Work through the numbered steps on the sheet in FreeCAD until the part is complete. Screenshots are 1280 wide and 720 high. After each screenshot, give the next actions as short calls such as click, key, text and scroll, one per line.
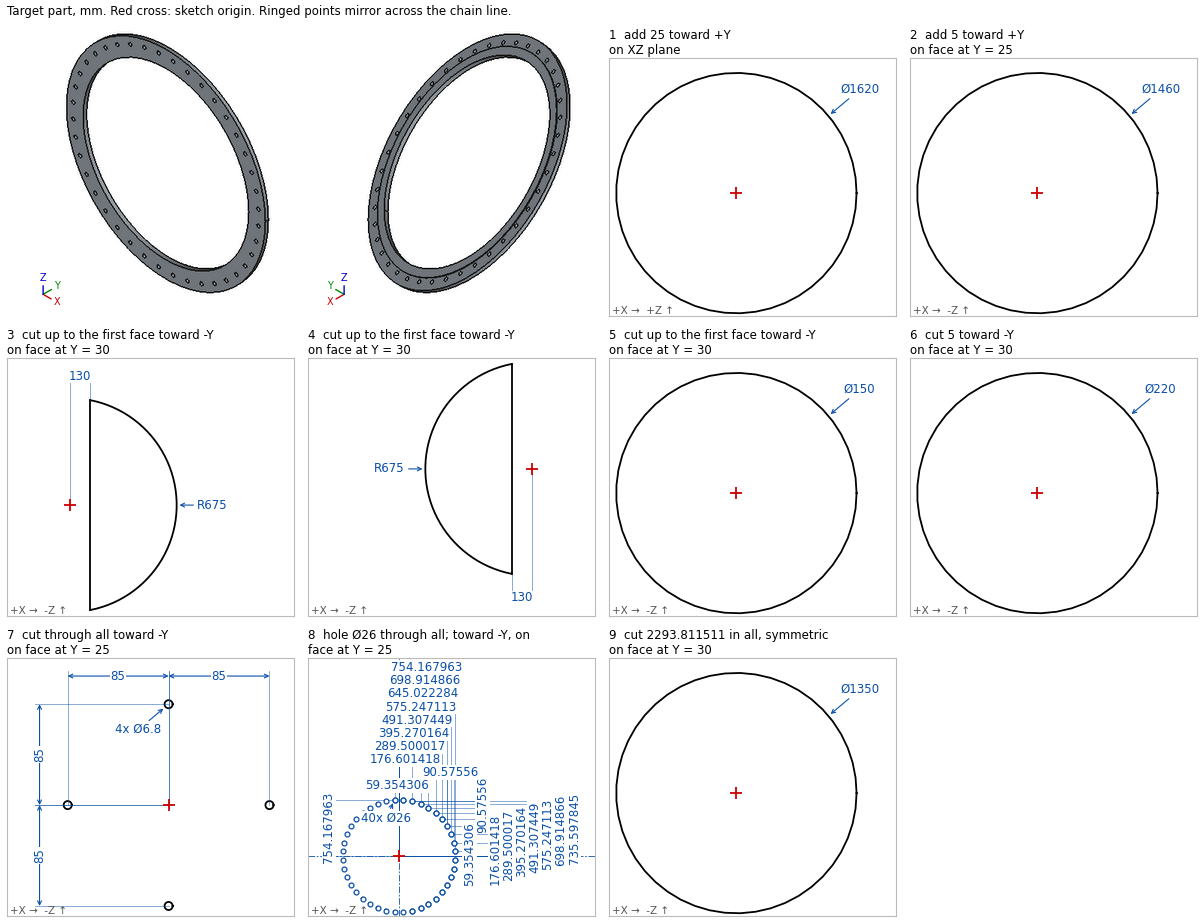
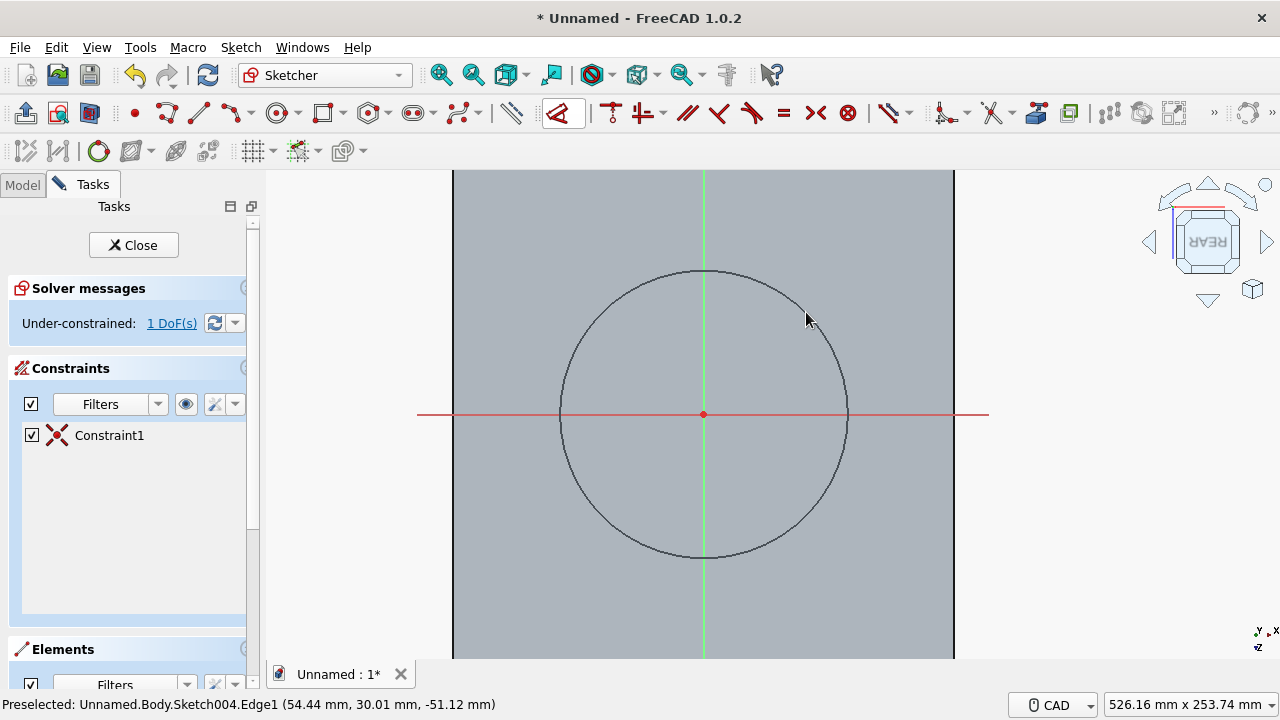
click(805, 312)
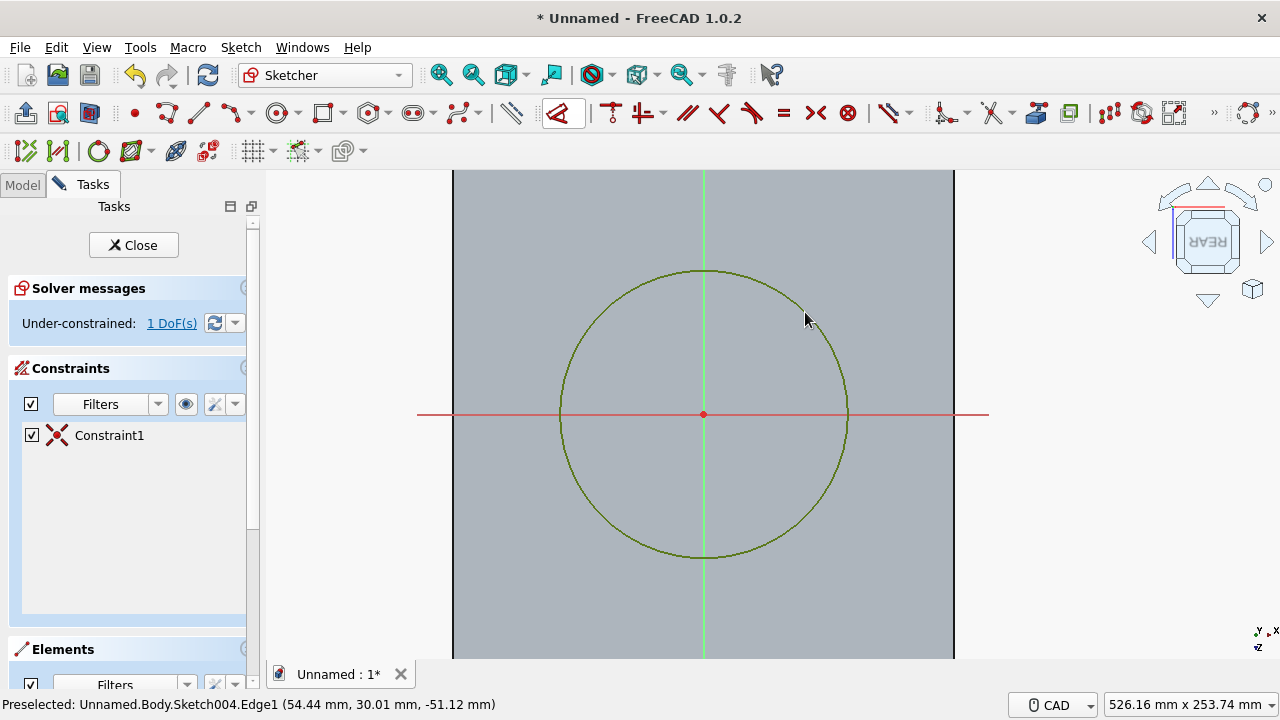
key(k)
key(o)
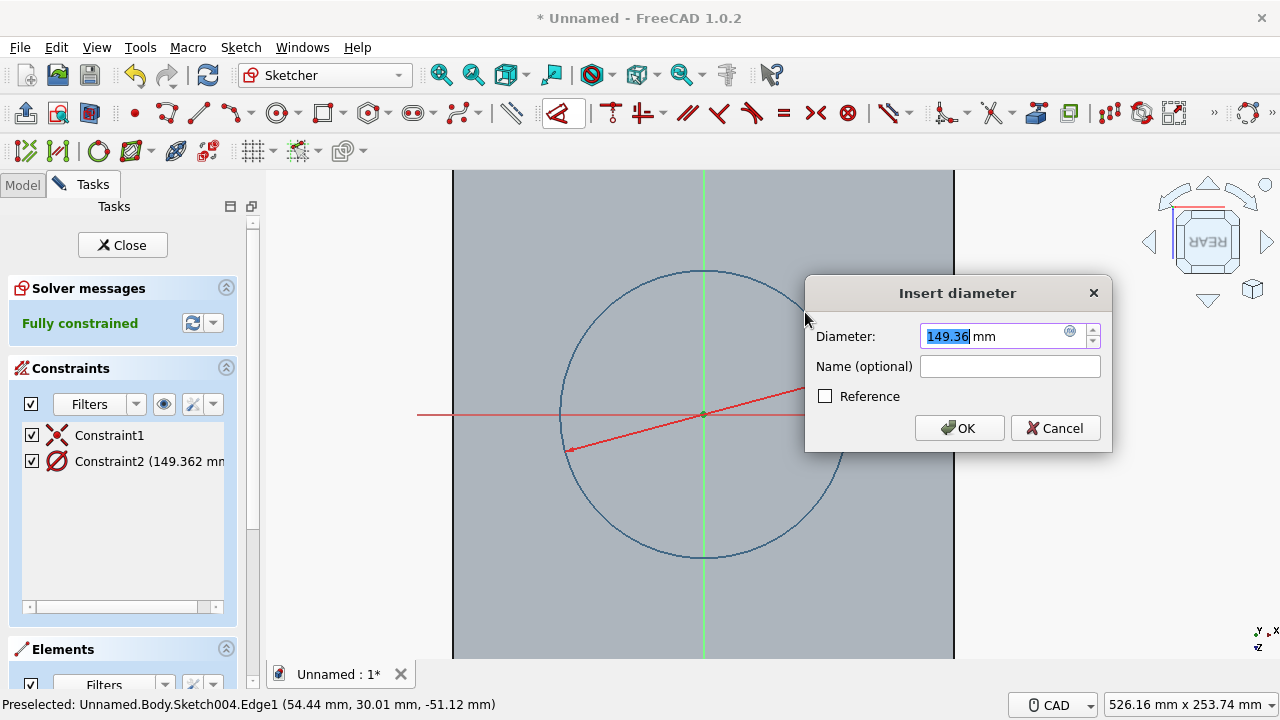
text(150)
key(Return)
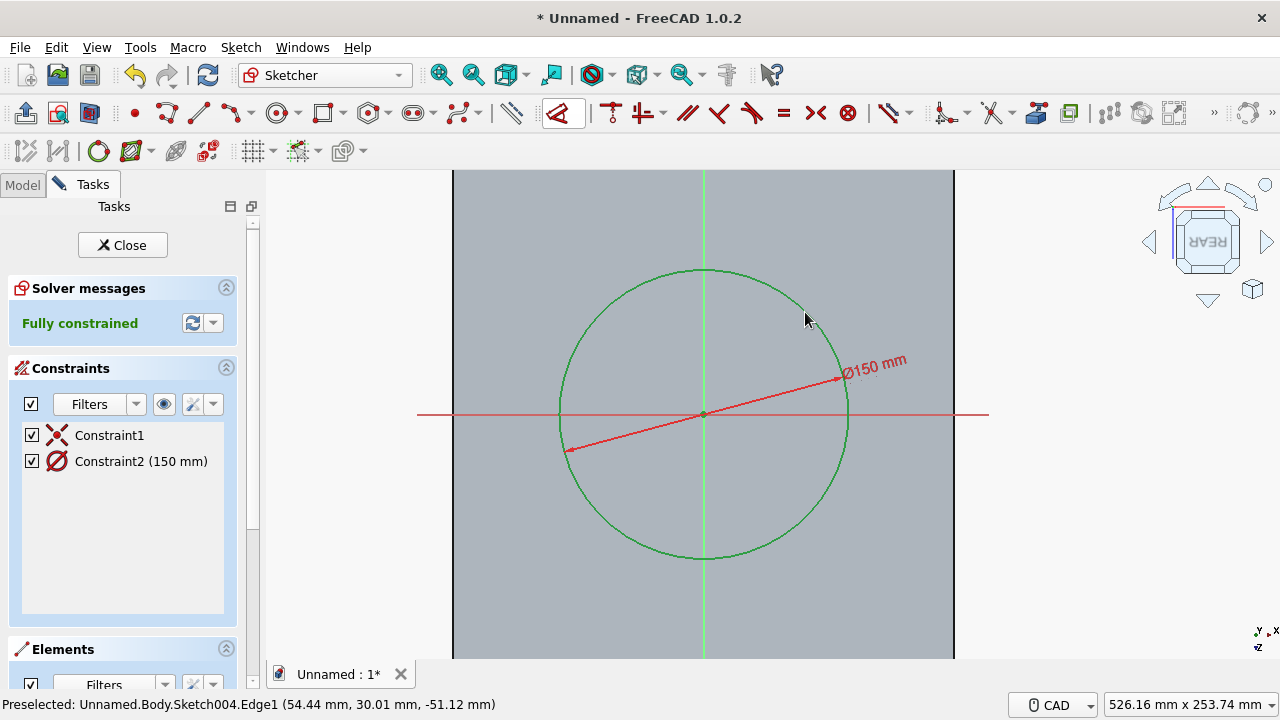
click(123, 245)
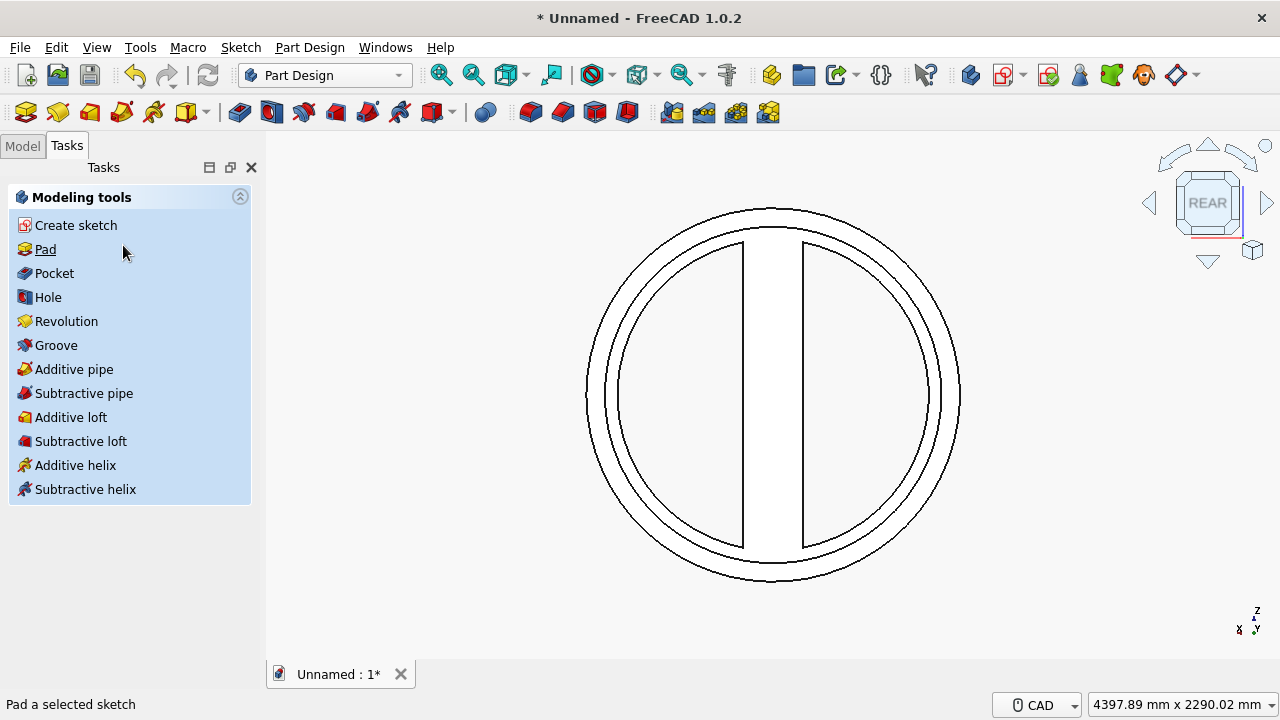
click(240, 112)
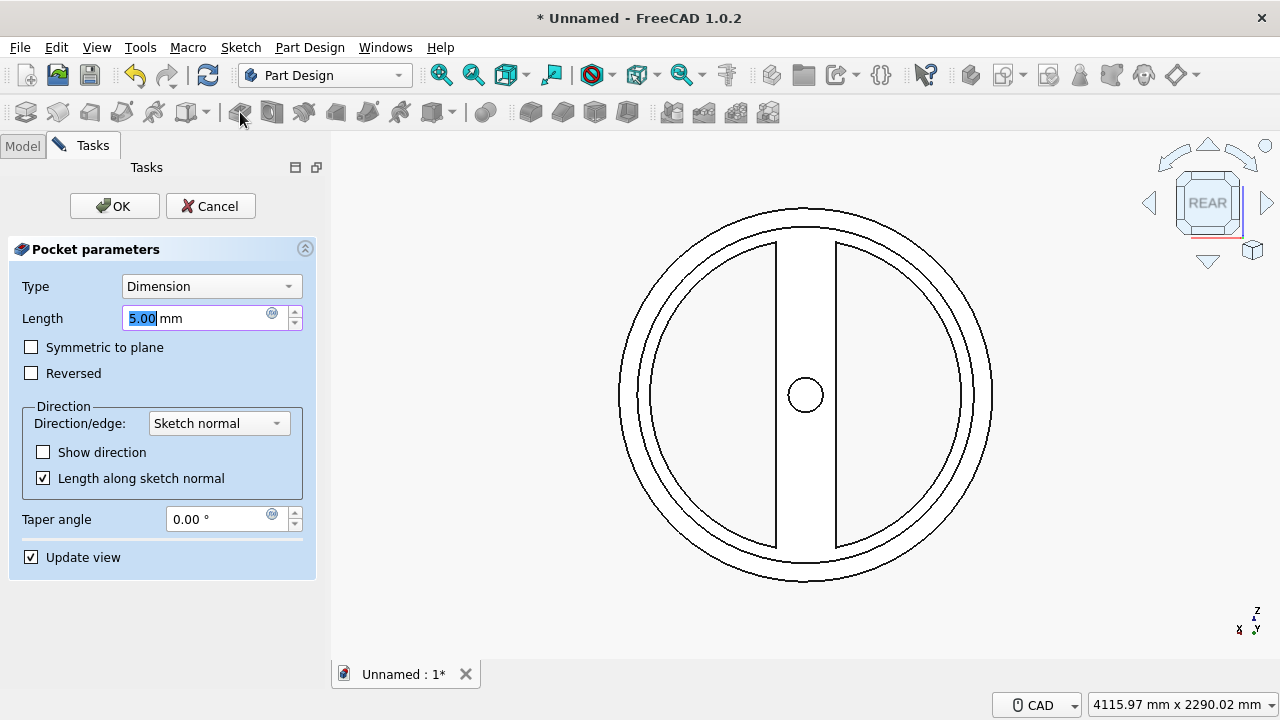
click(212, 286)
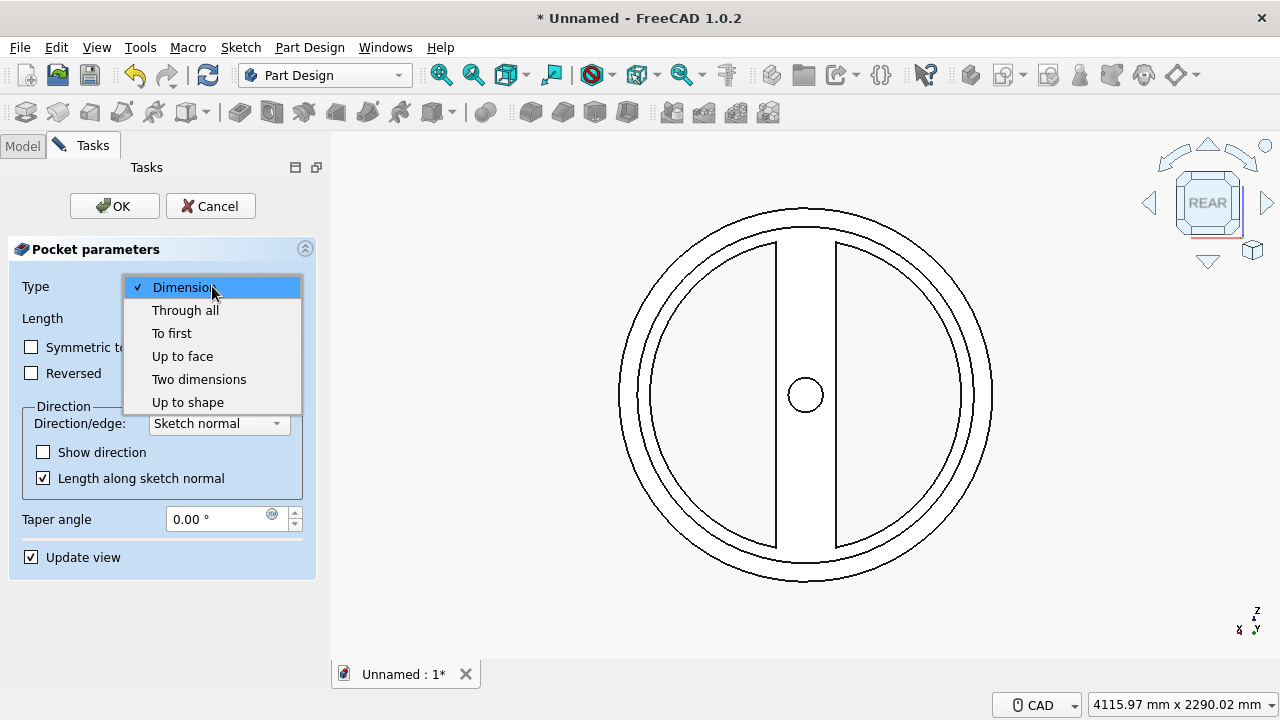
click(212, 334)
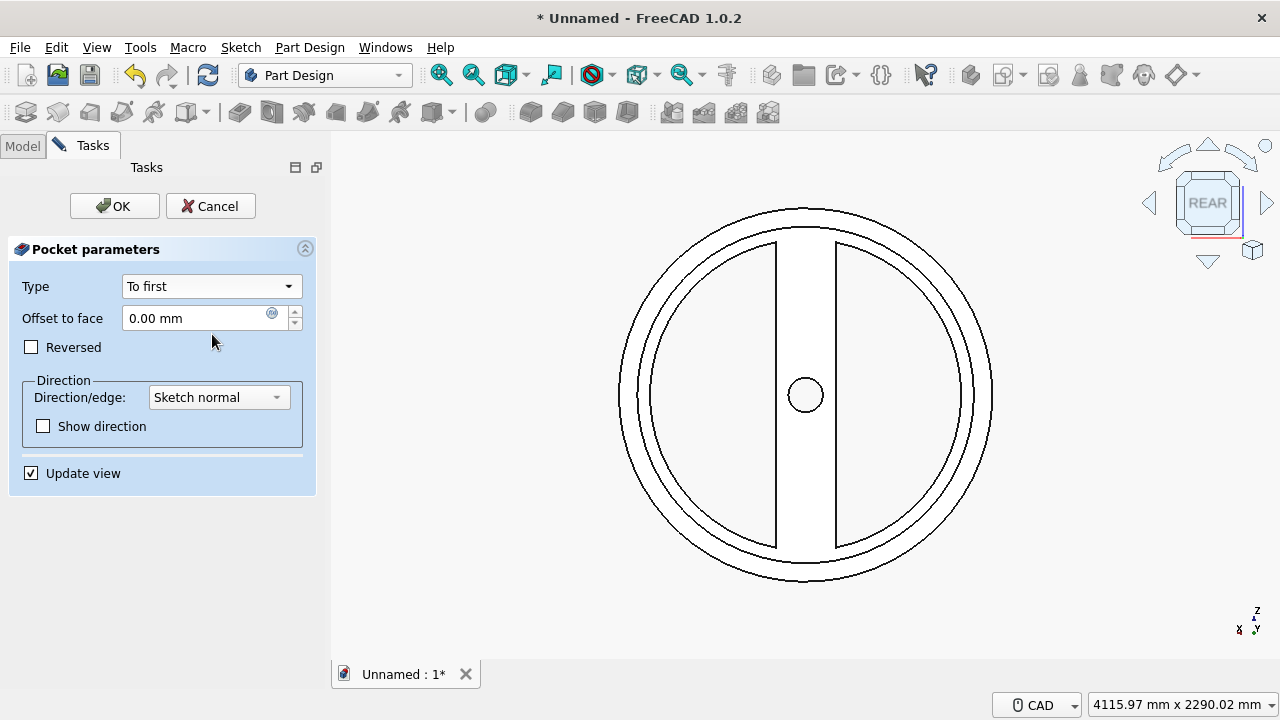
click(115, 206)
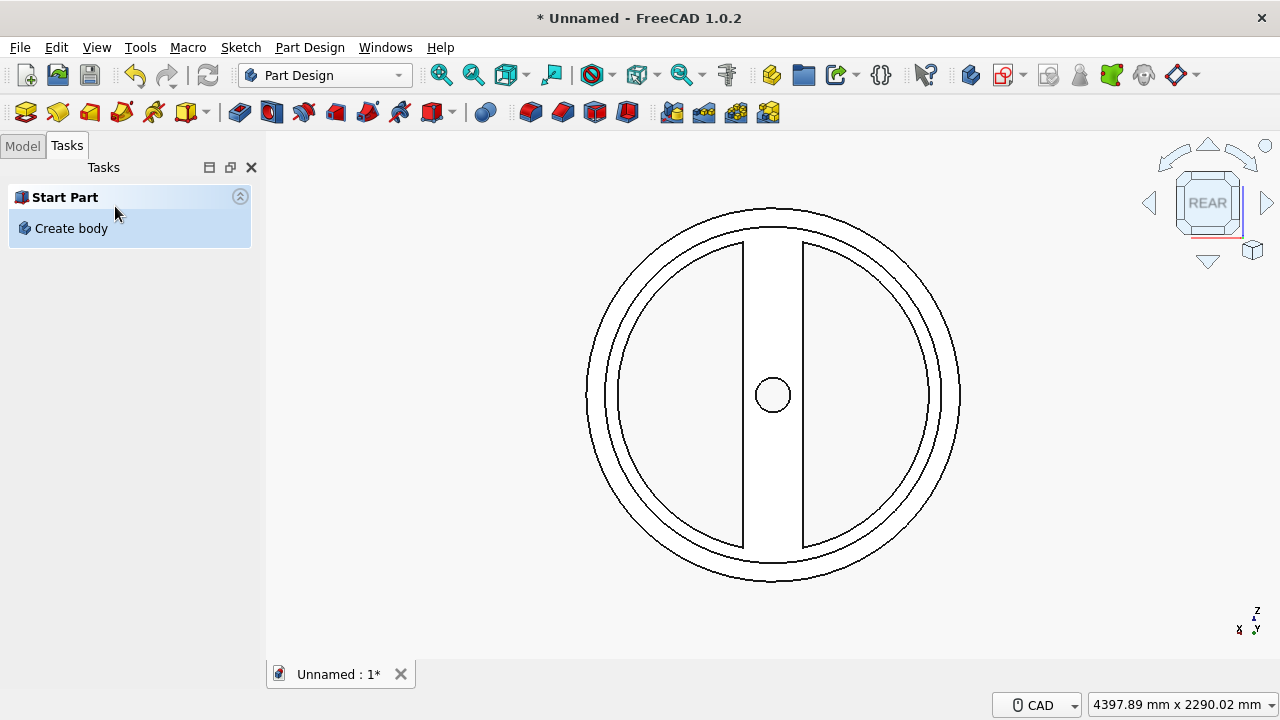
click(773, 490)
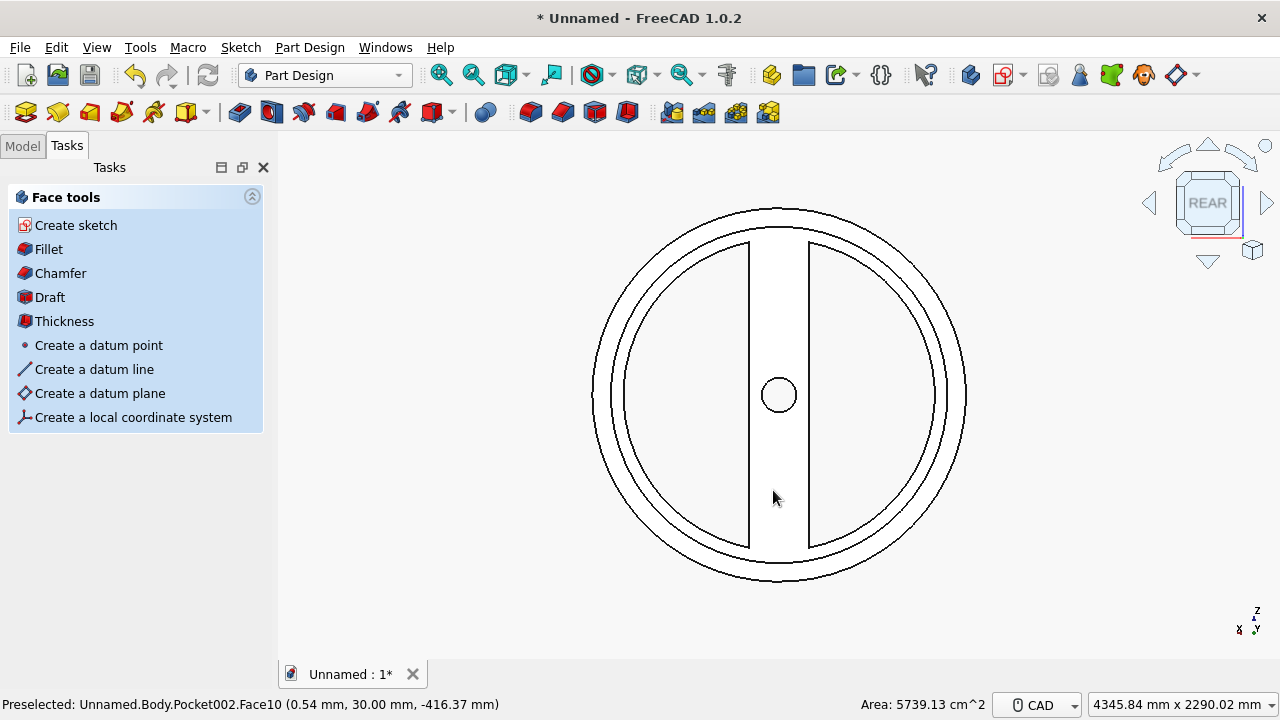
click(1004, 76)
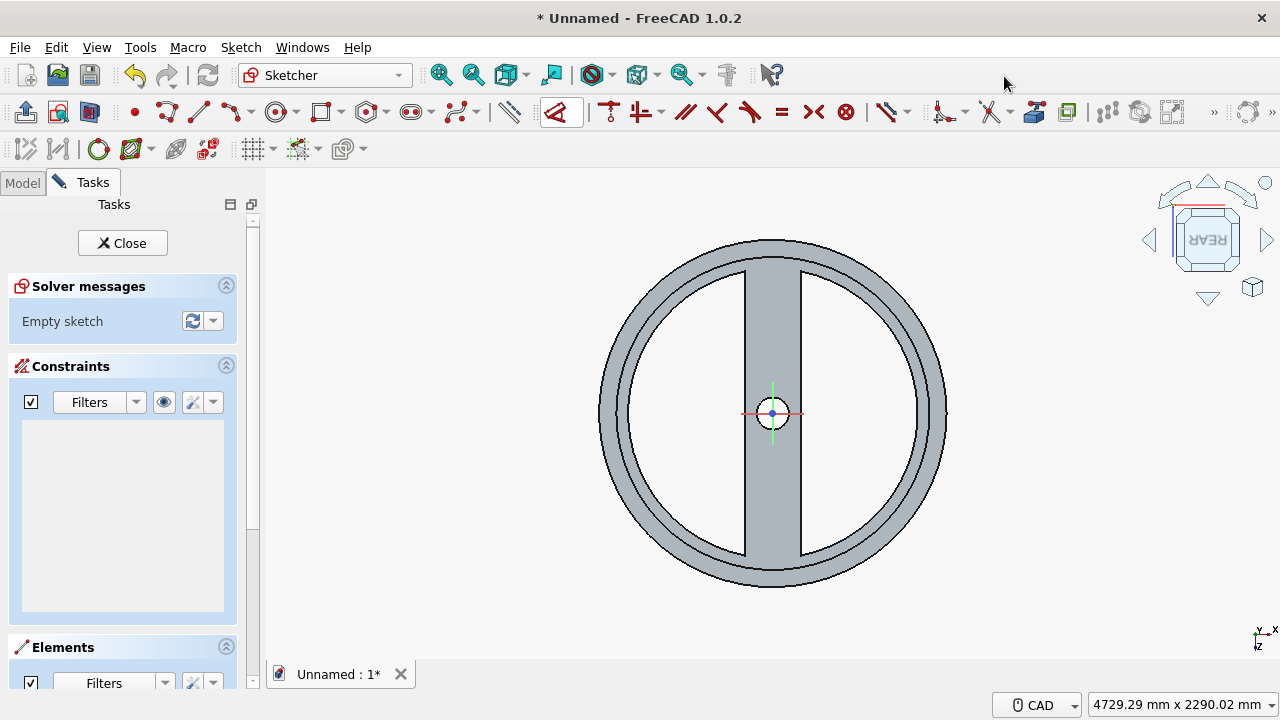
scroll(786, 413, up, 9)